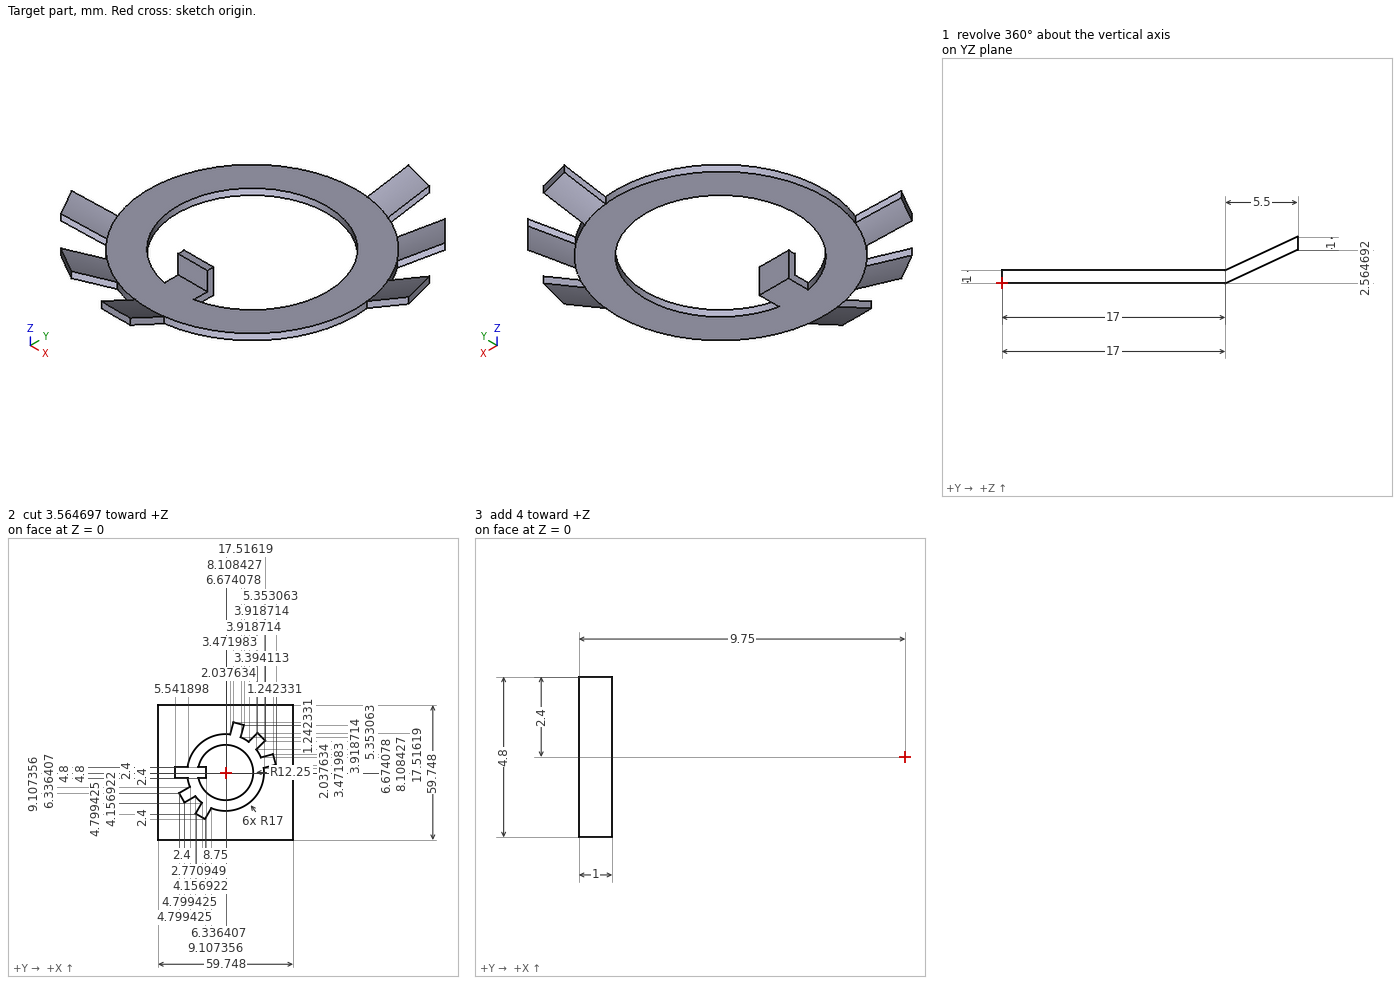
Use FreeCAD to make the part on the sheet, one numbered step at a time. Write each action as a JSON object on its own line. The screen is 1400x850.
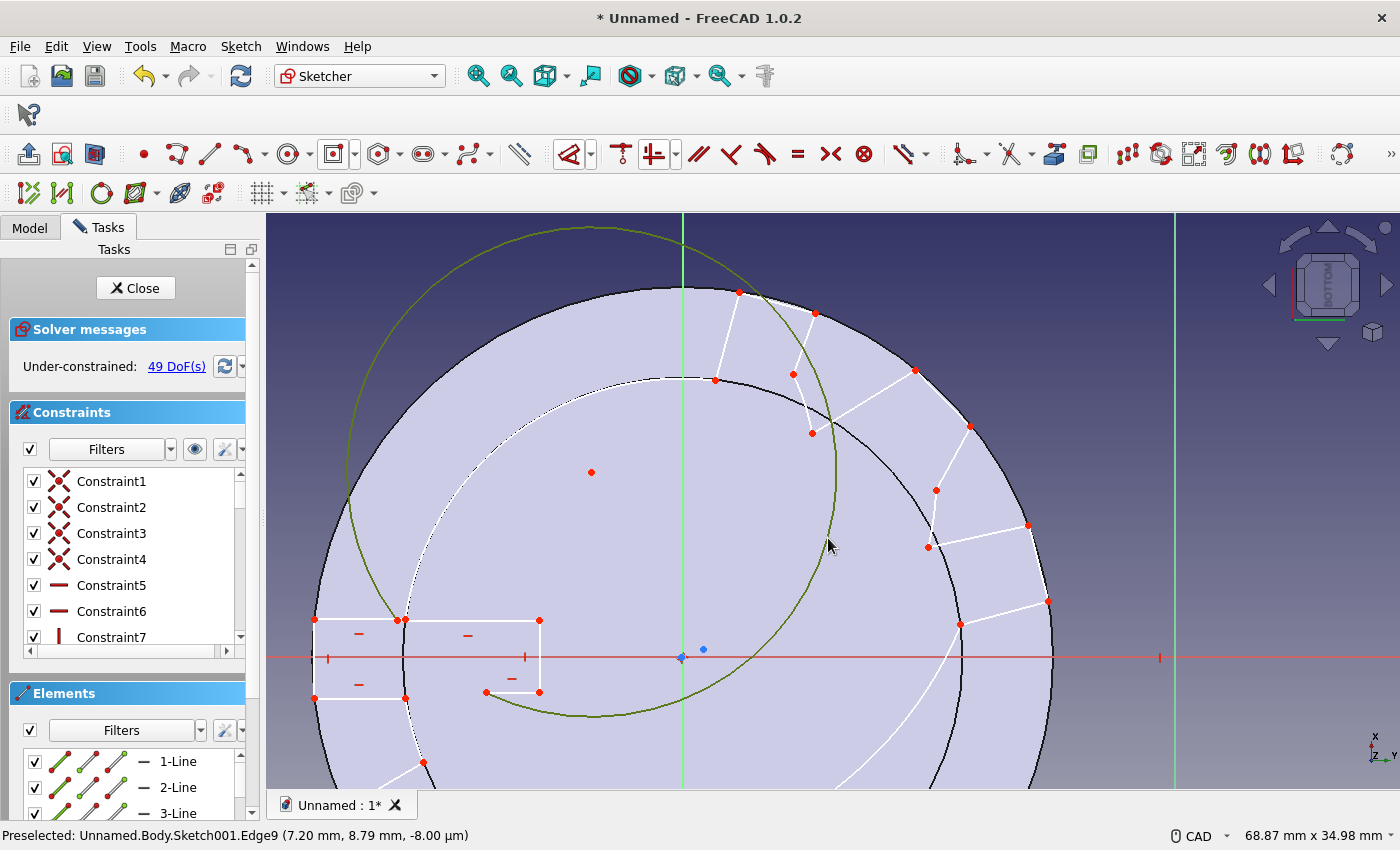
{"action": "left_click", "coordinate": [587, 395]}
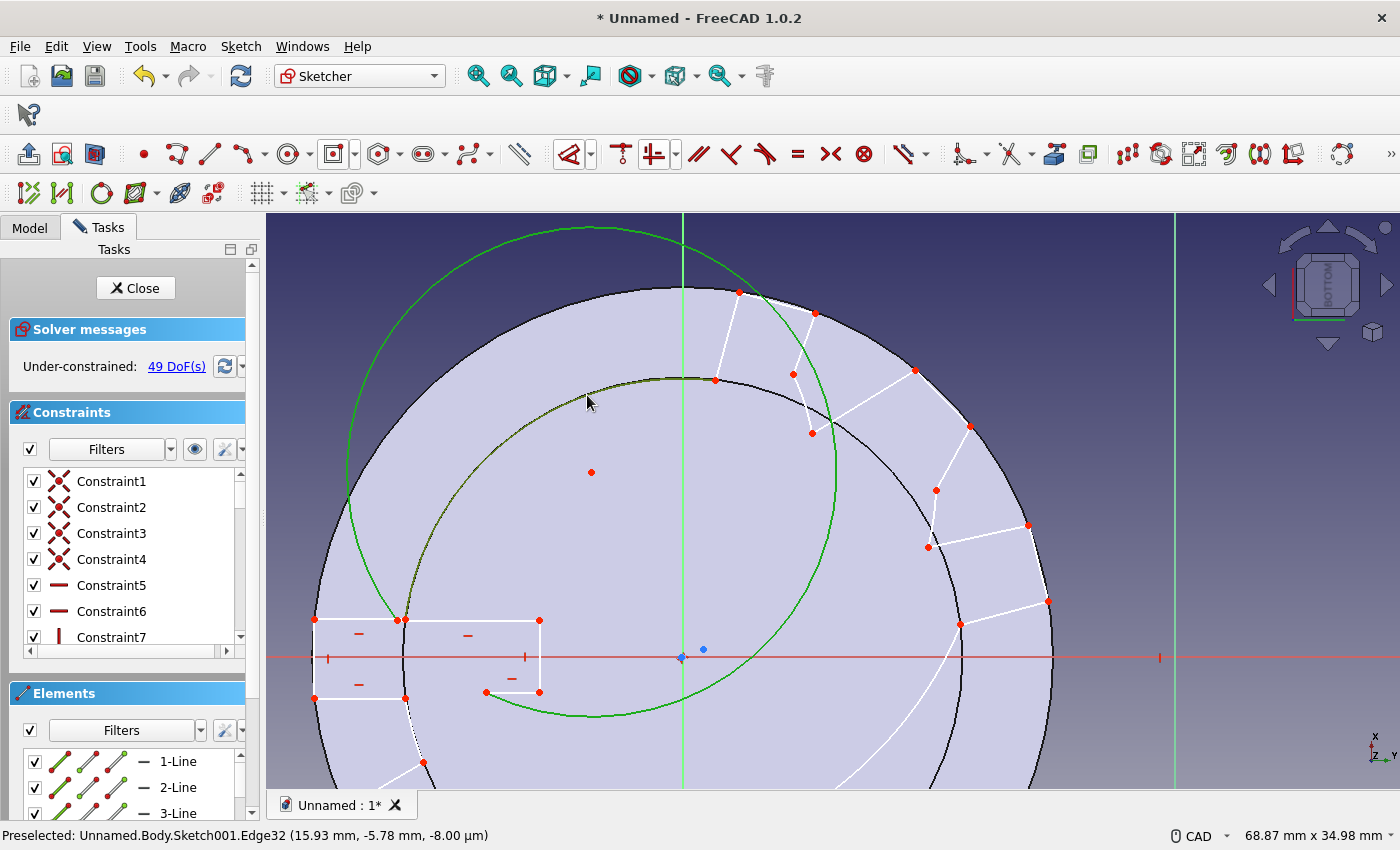
{"action": "left_click", "coordinate": [621, 154]}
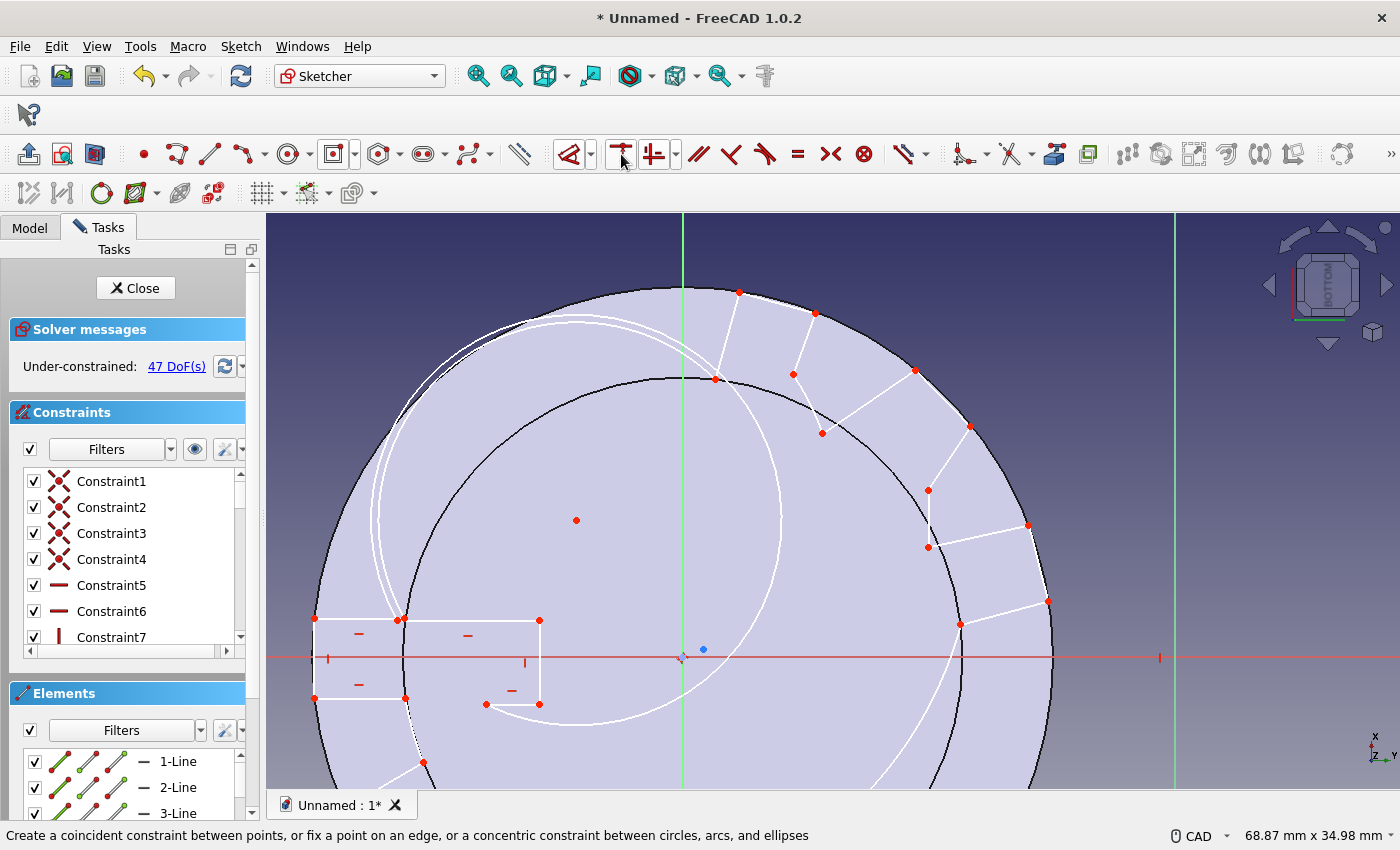
{"action": "left_click", "coordinate": [771, 585]}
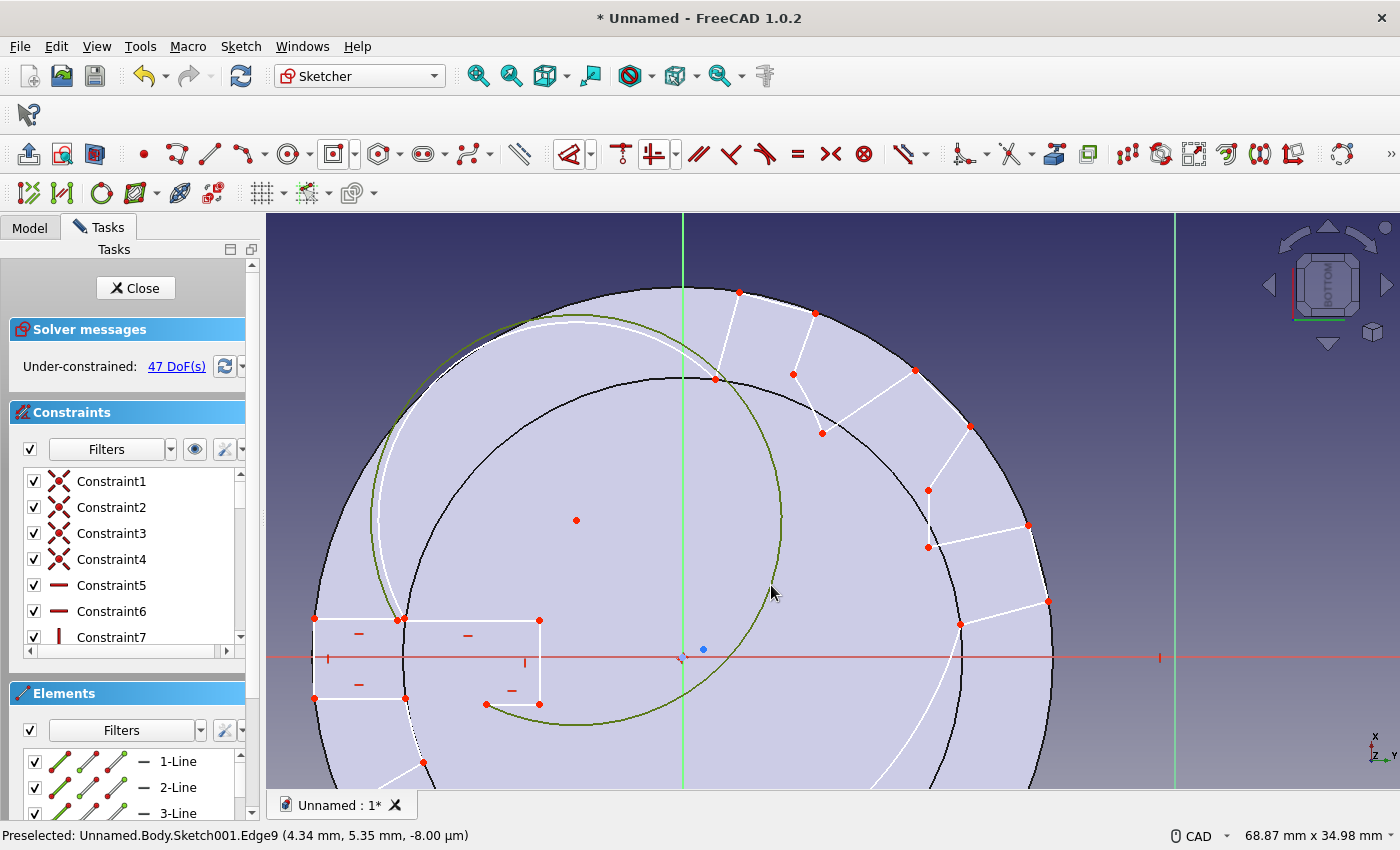
{"action": "left_click", "coordinate": [409, 718]}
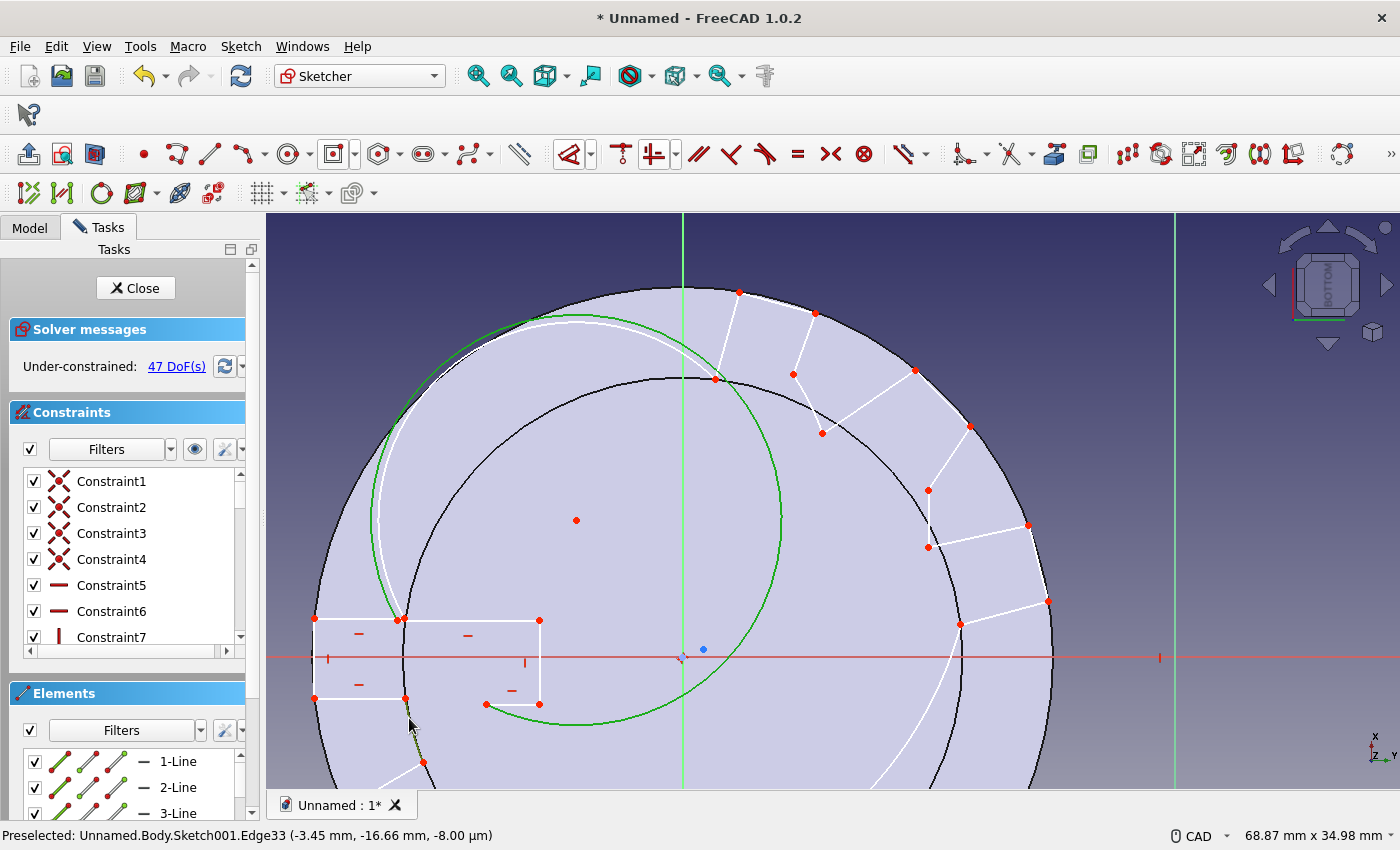
{"action": "left_click", "coordinate": [621, 154]}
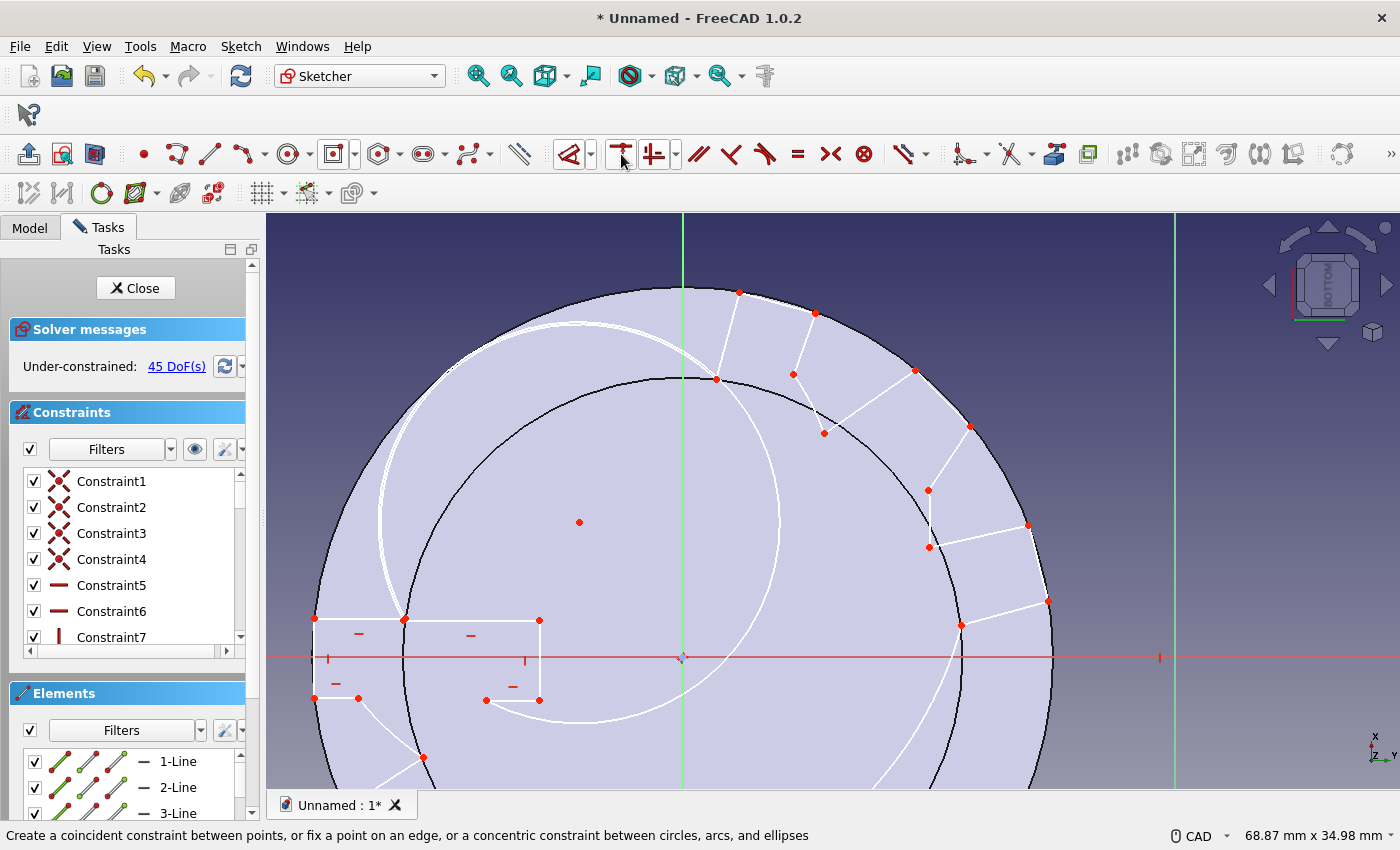
{"action": "left_click_drag", "start_coordinate": [569, 513], "coordinate": [693, 667]}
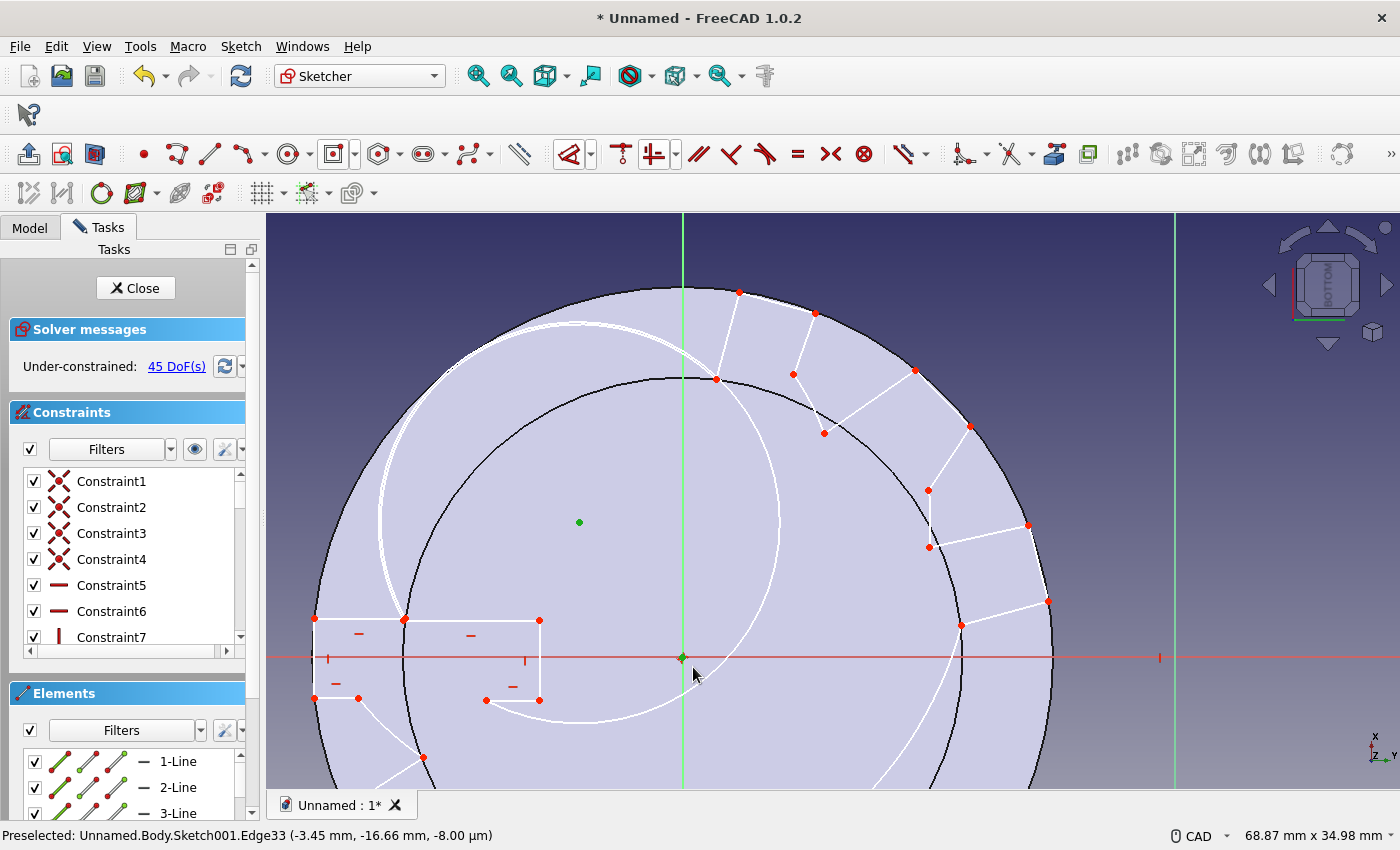
{"action": "left_click", "coordinate": [621, 154]}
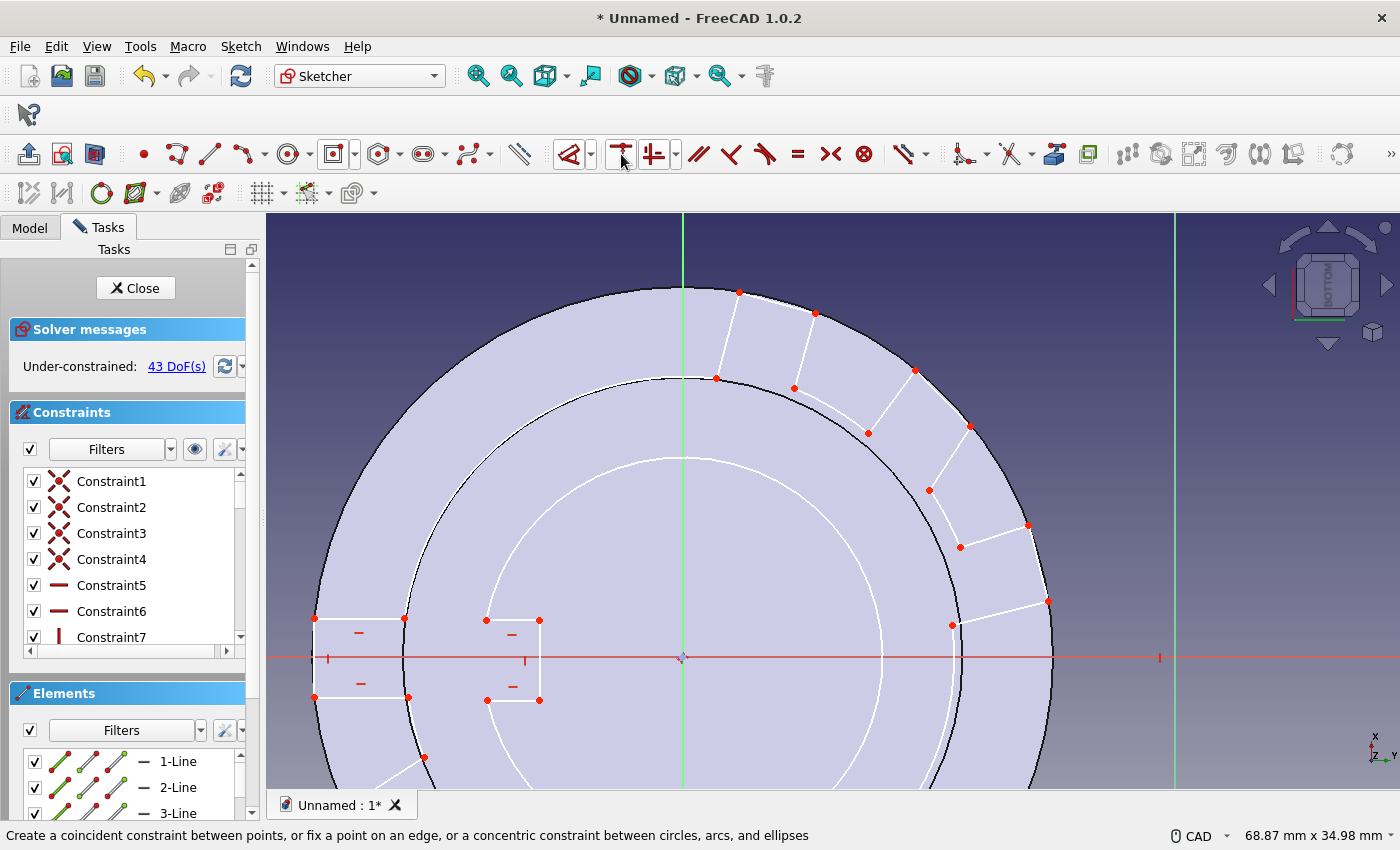
{"action": "scroll", "coordinate": [812, 410], "scroll_direction": "down", "scroll_amount": 5}